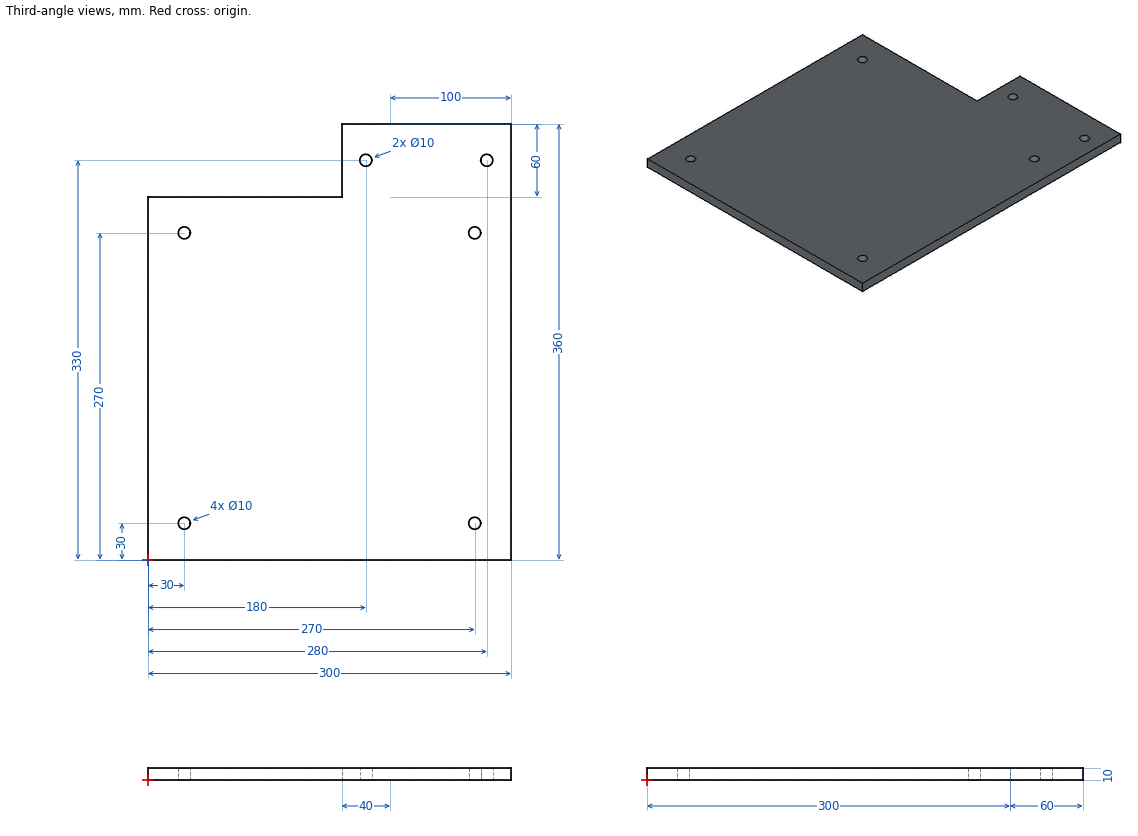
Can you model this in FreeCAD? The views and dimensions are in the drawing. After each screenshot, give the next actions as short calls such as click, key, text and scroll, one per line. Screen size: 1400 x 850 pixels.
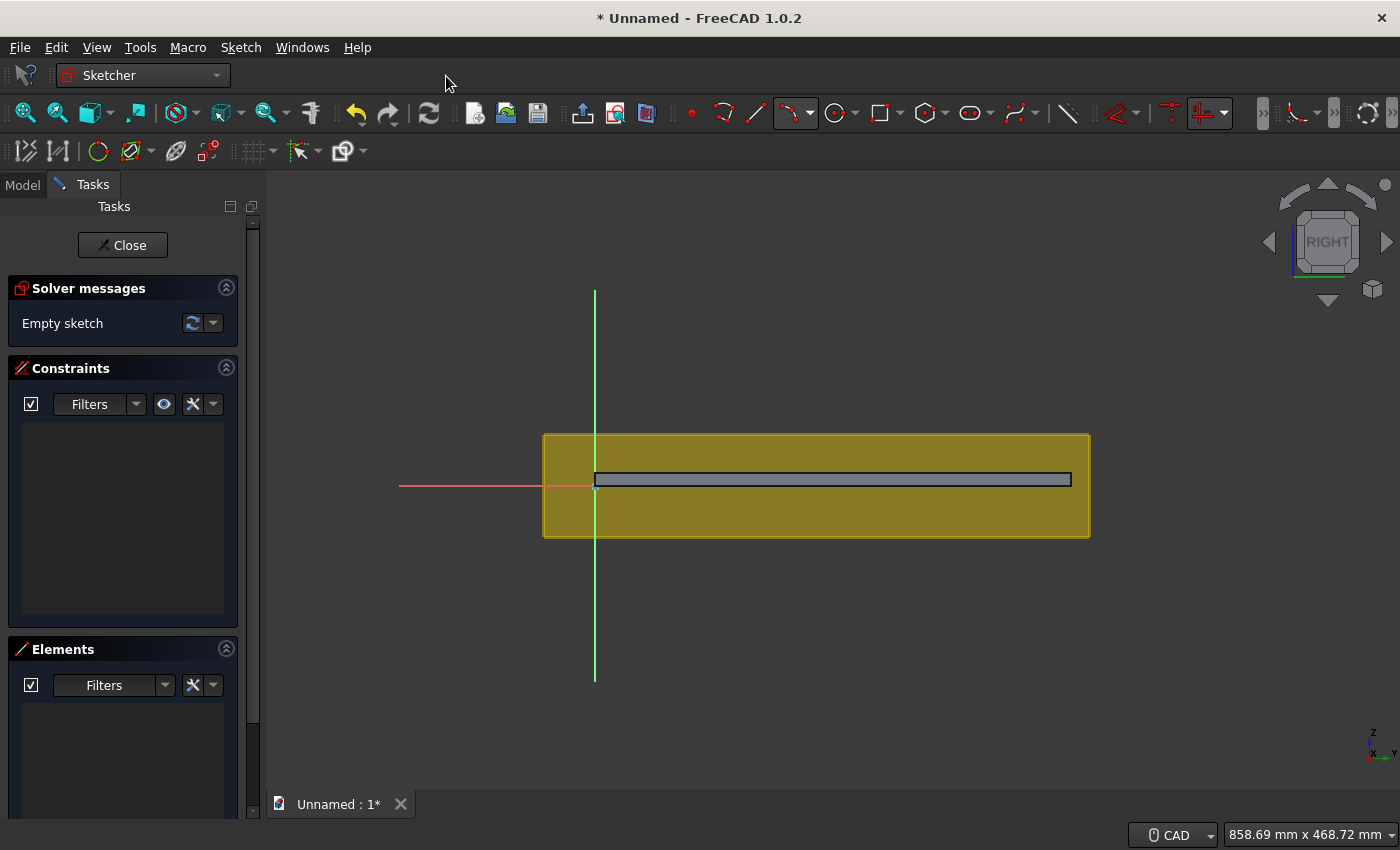
click(648, 114)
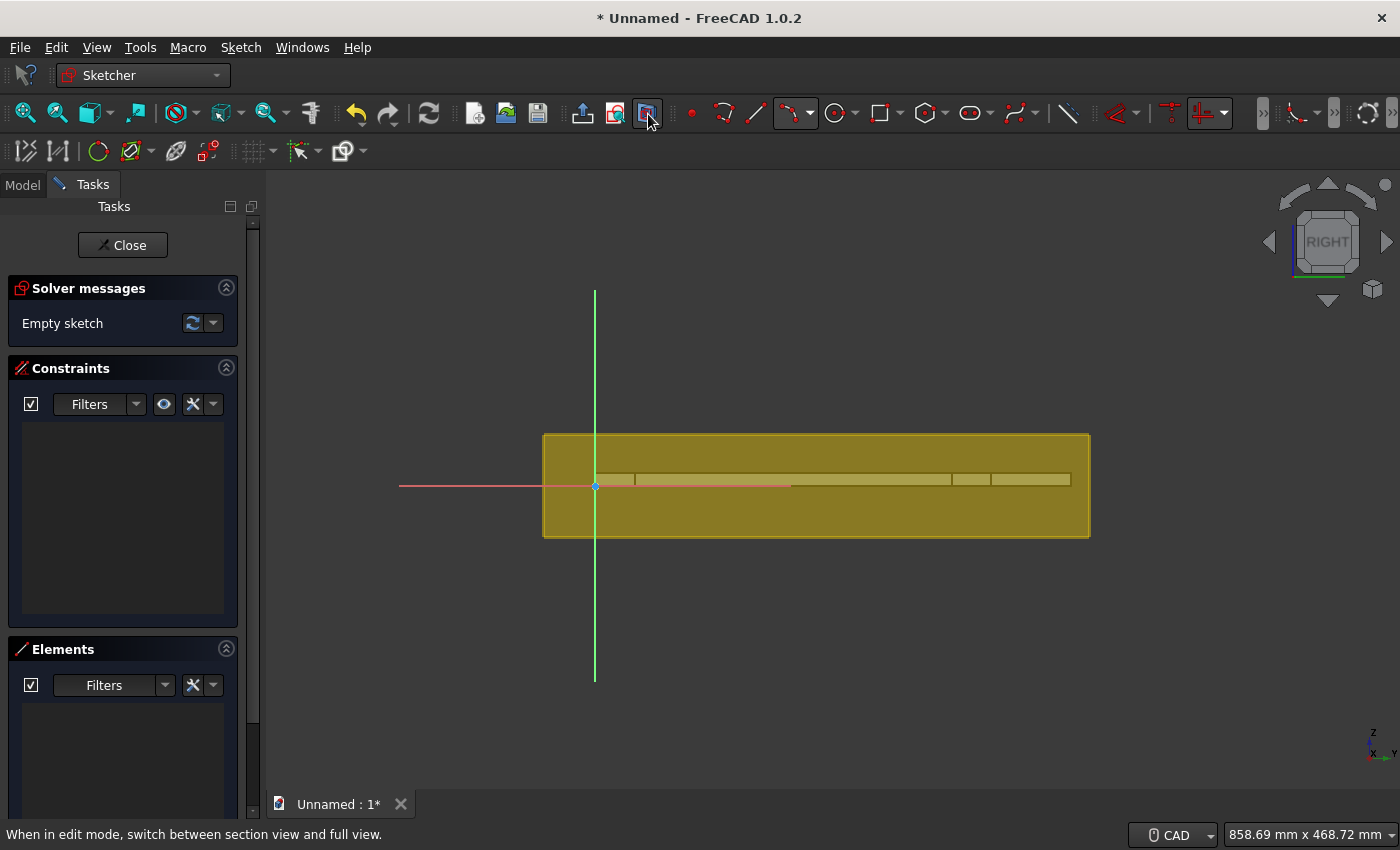
scroll(1064, 479, up, 11)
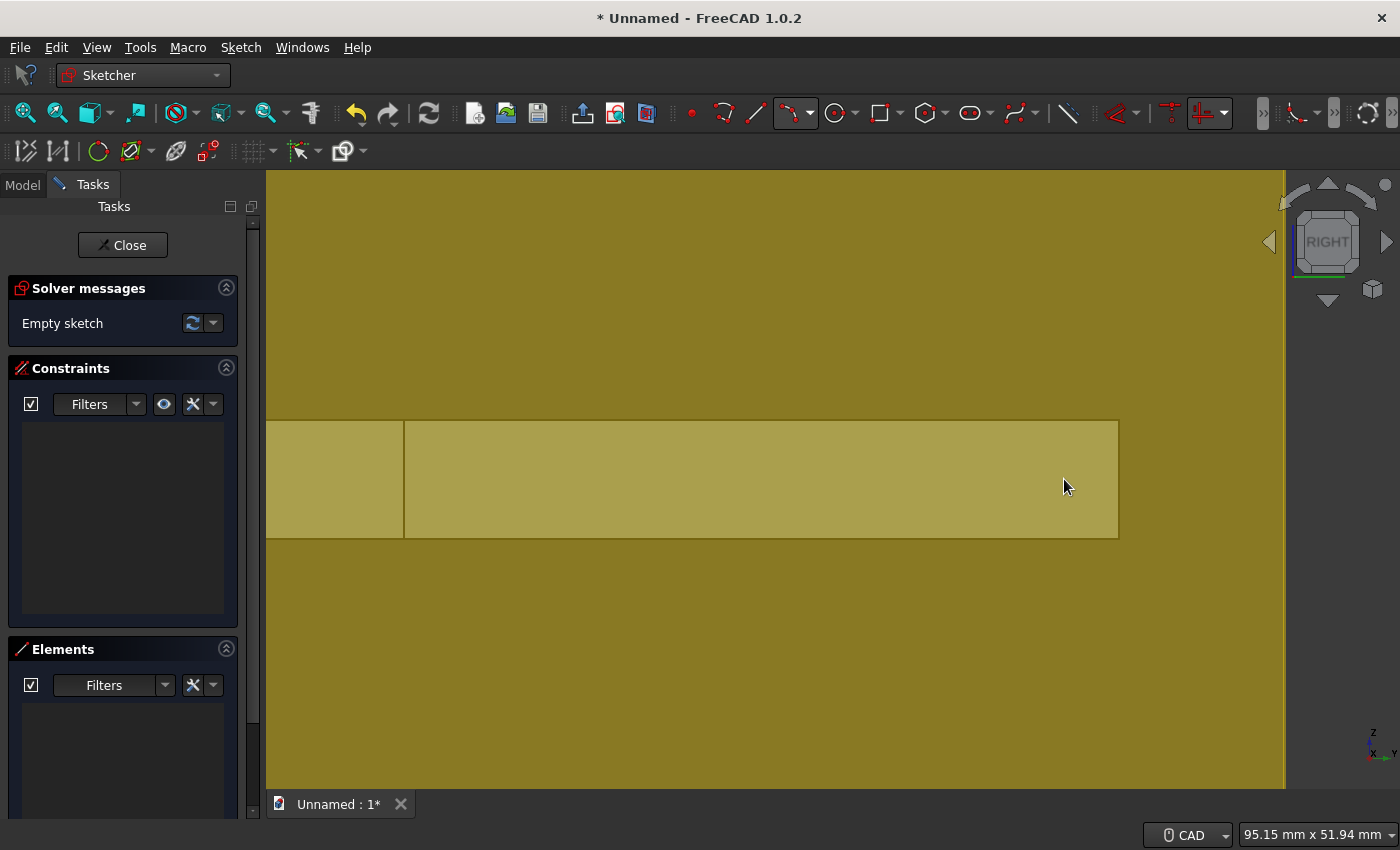
click(880, 114)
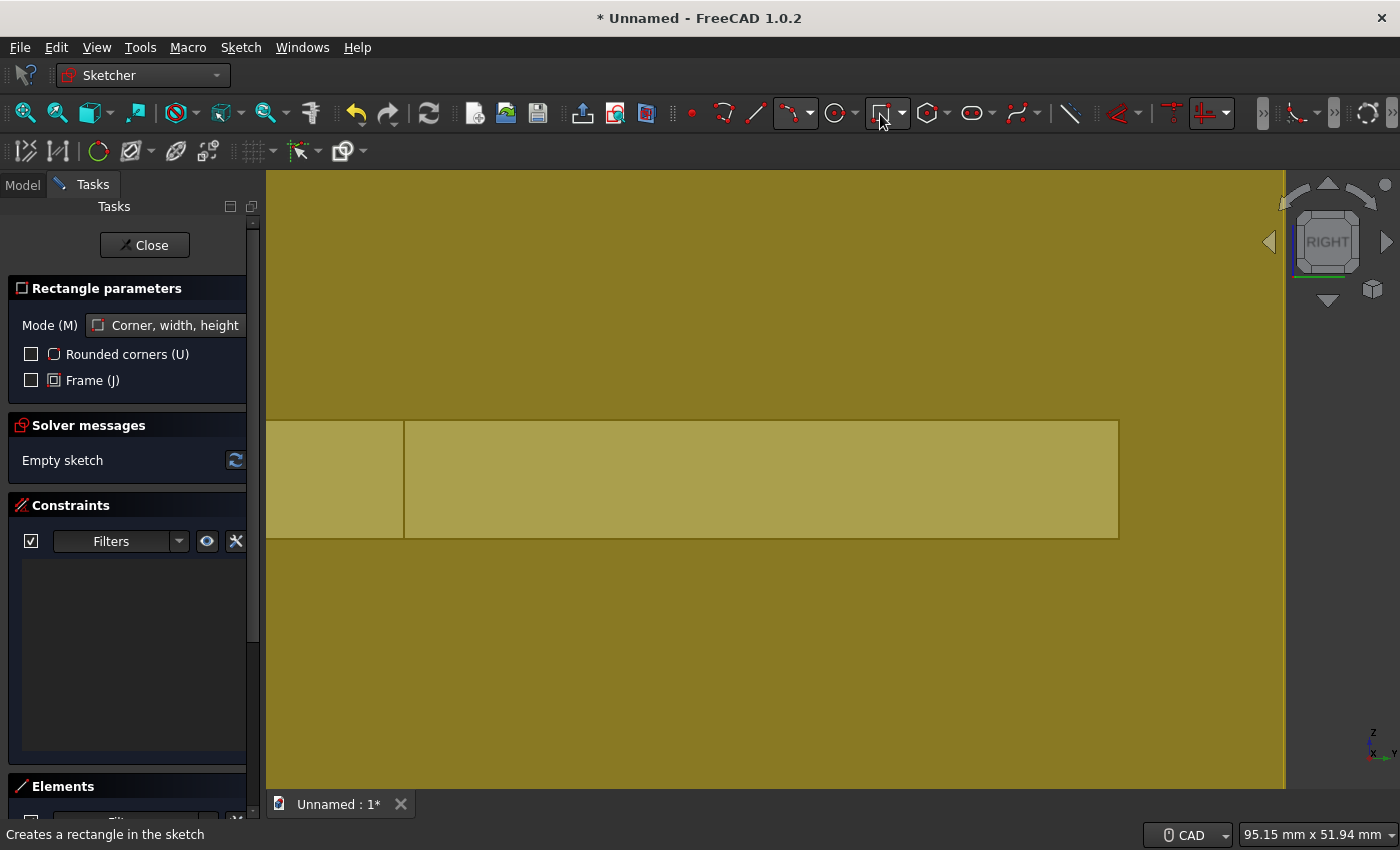
click(404, 420)
click(1119, 539)
key(Escape)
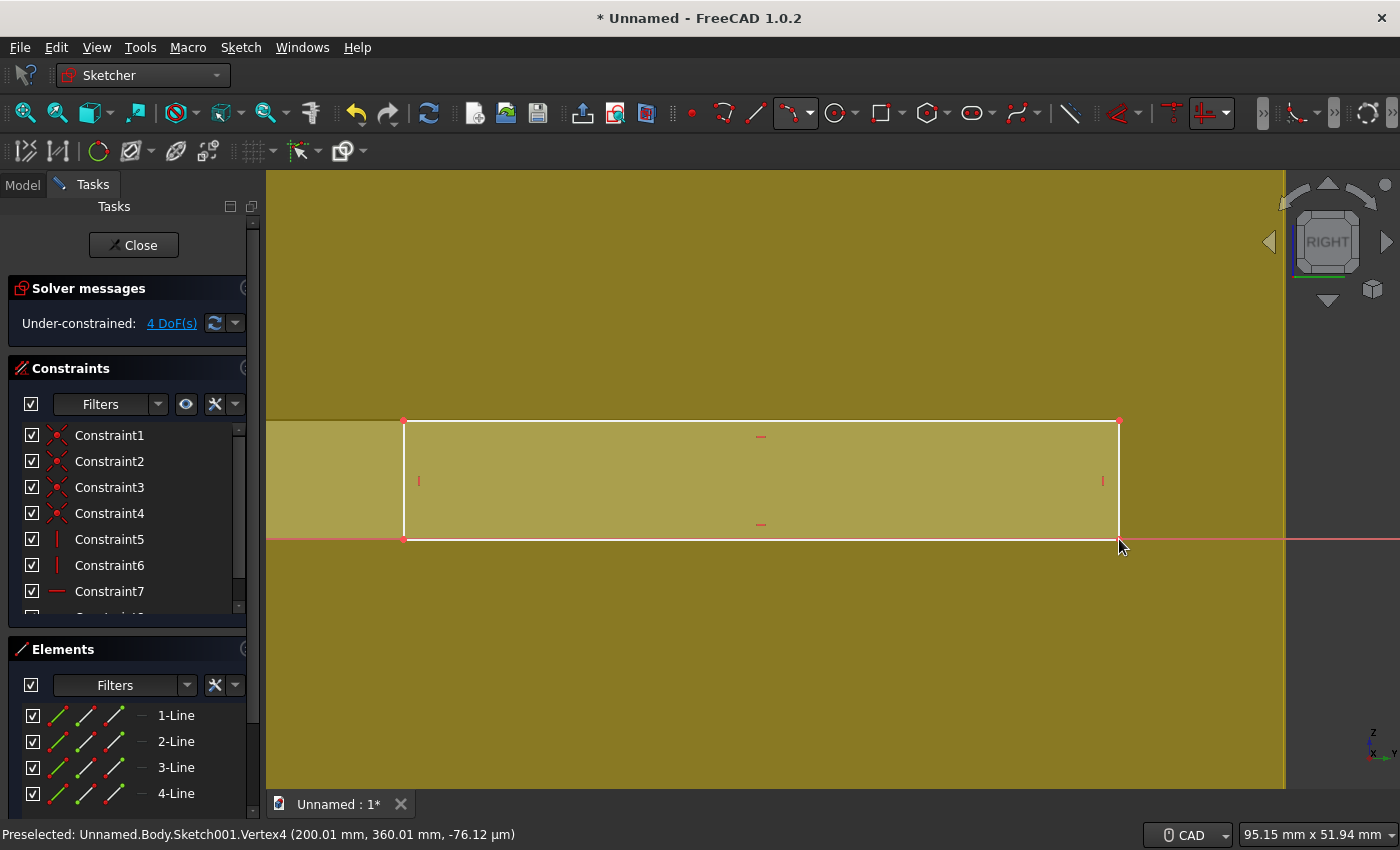
click(404, 540)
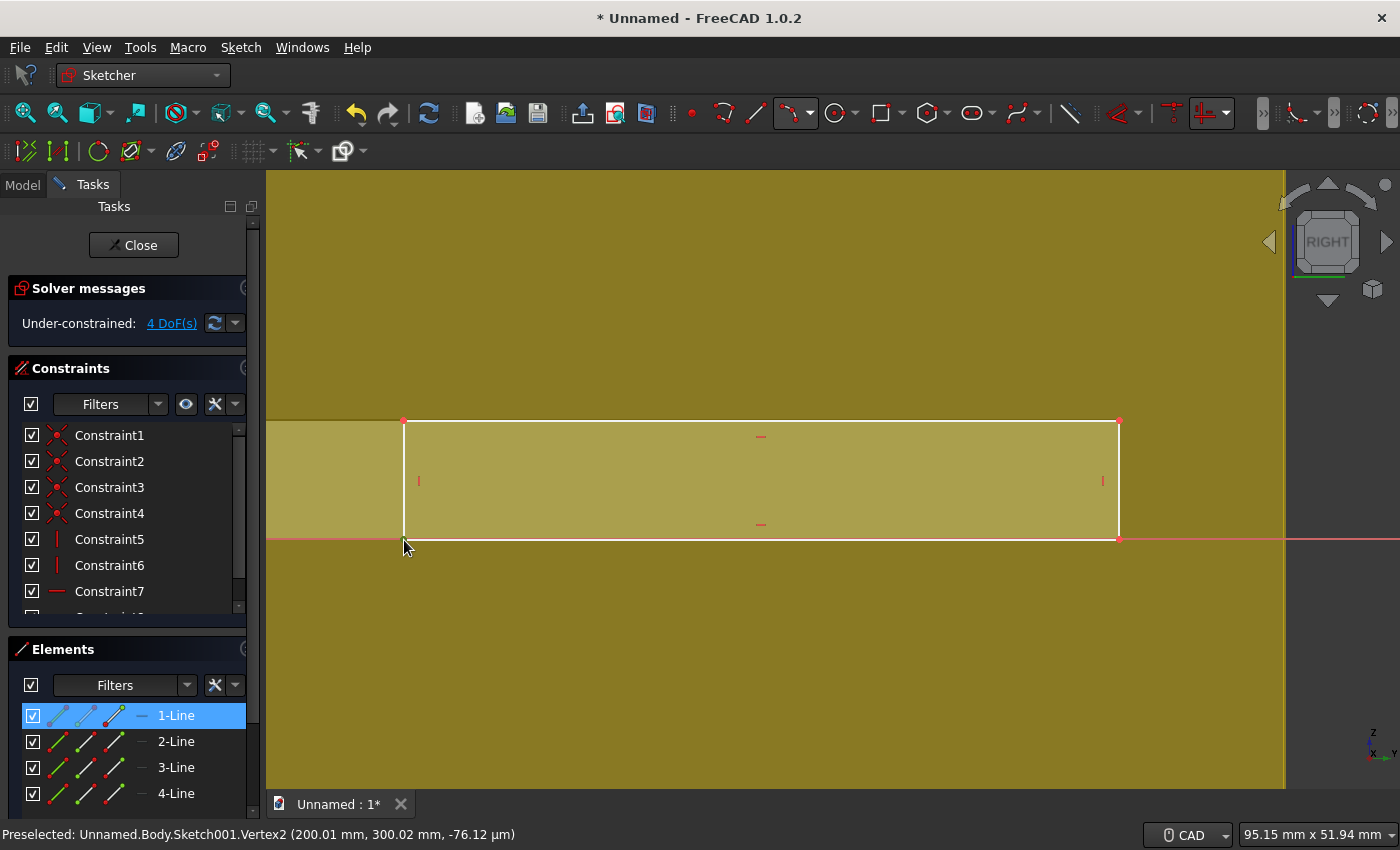
click(361, 539)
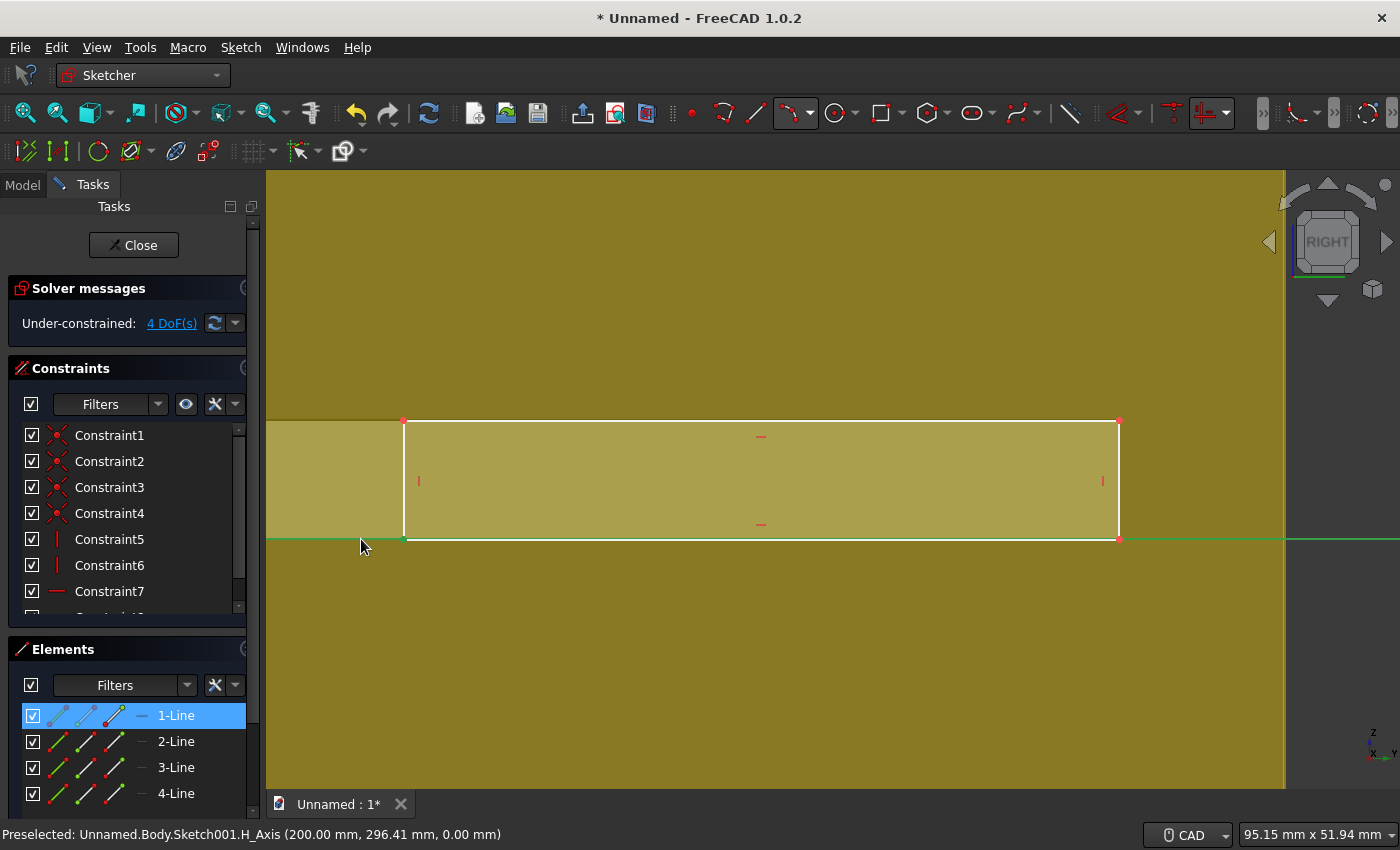
click(1172, 114)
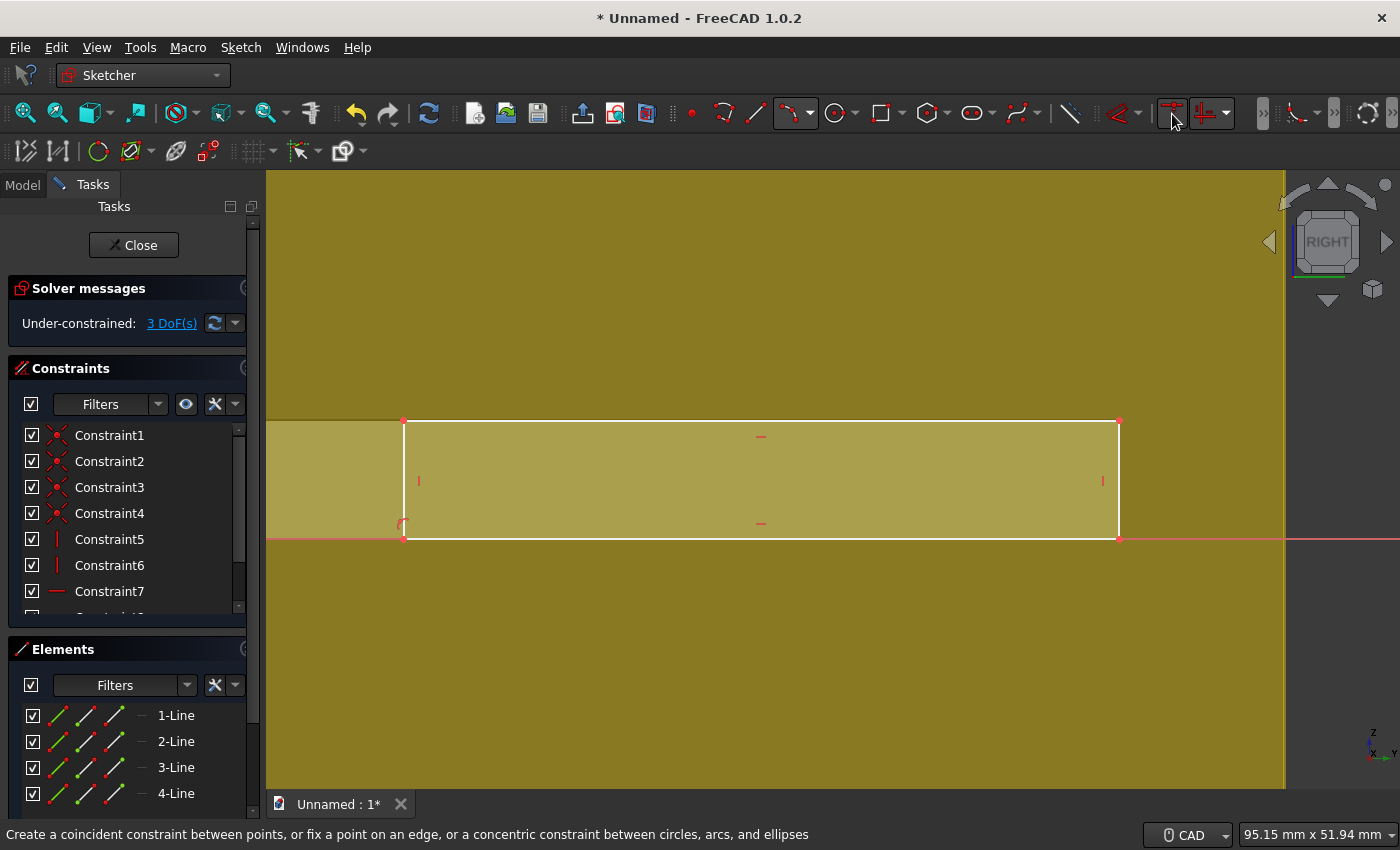
click(1118, 114)